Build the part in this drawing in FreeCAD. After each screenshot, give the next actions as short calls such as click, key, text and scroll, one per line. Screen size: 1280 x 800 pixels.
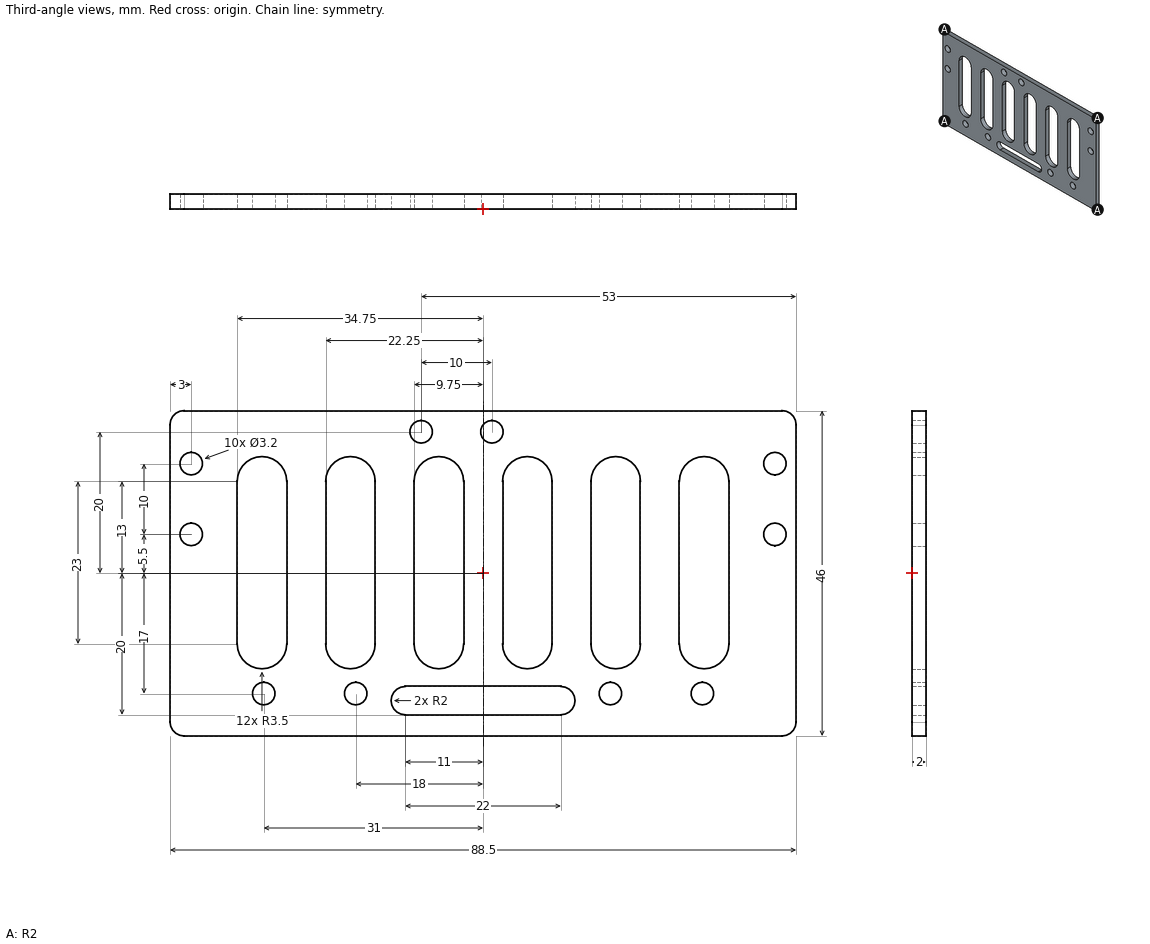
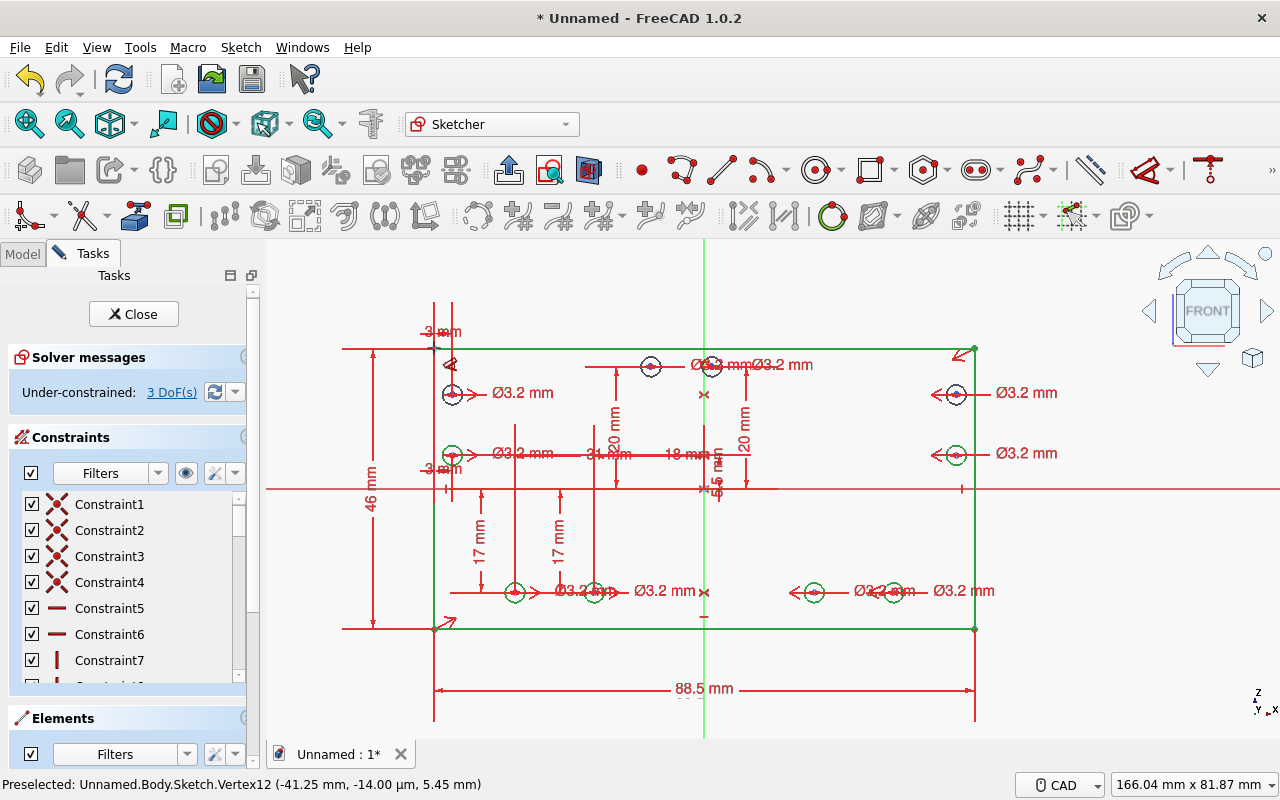
click(975, 349)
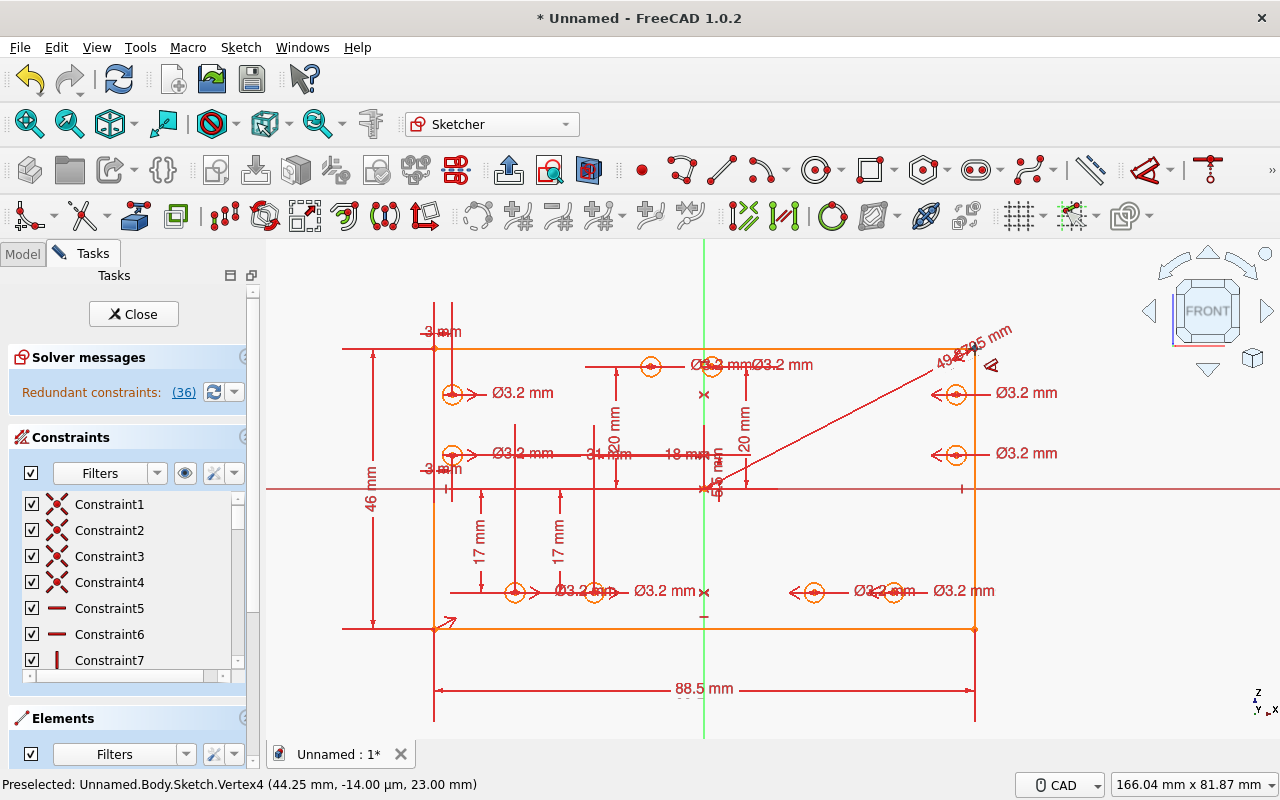
click(651, 367)
click(813, 315)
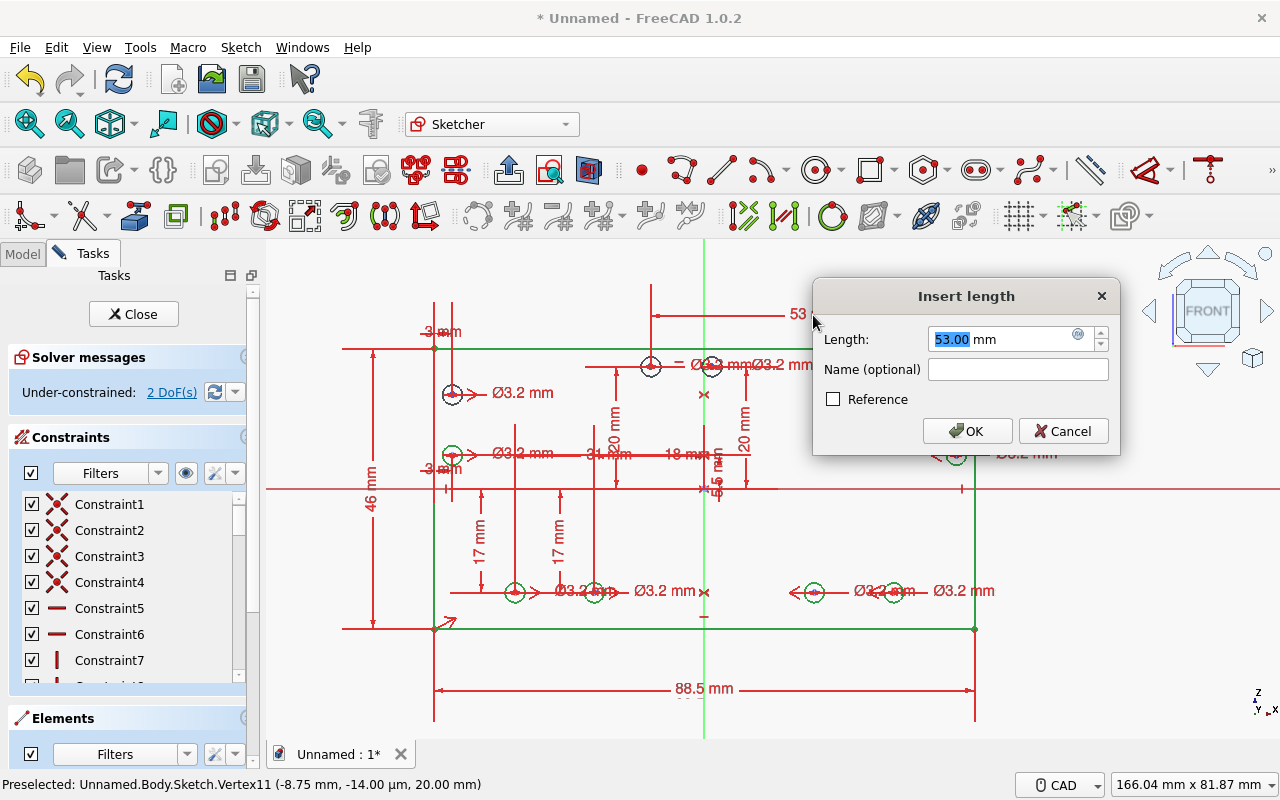
text(53)
key(Return)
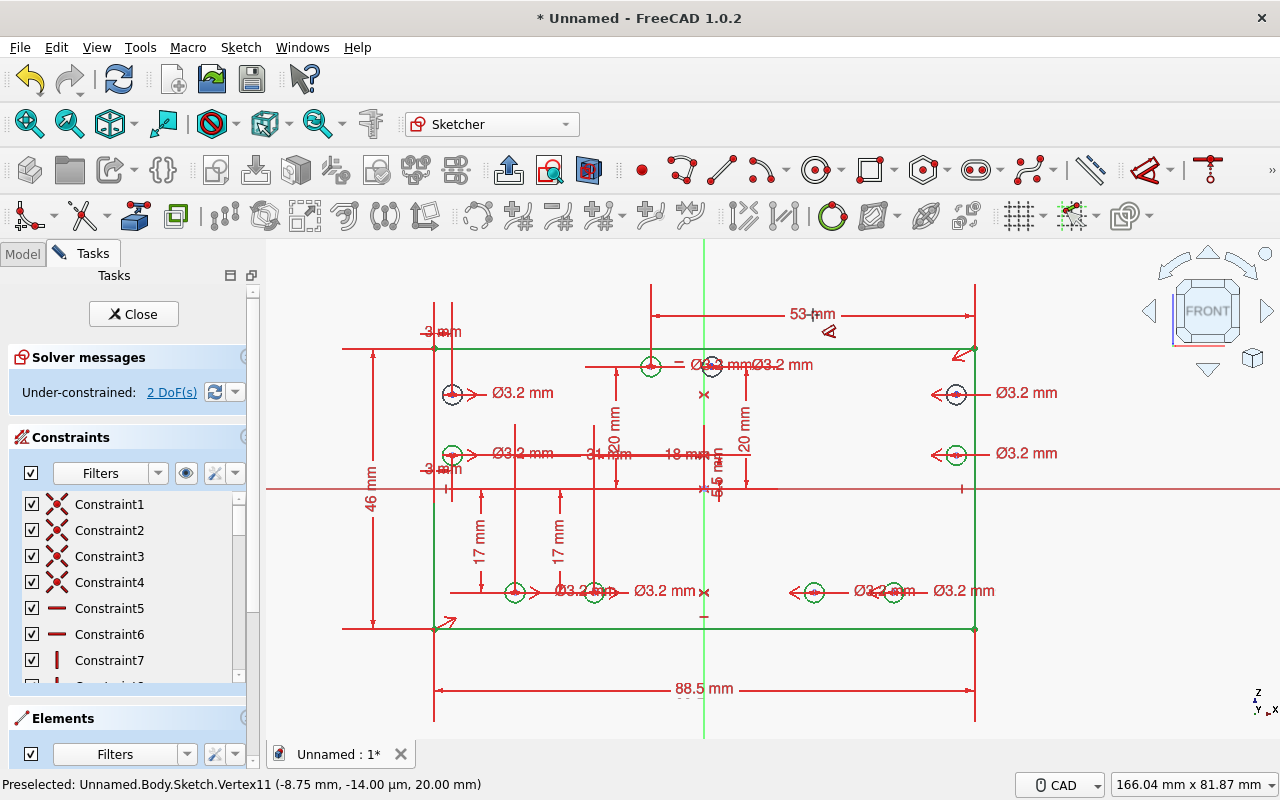
click(452, 395)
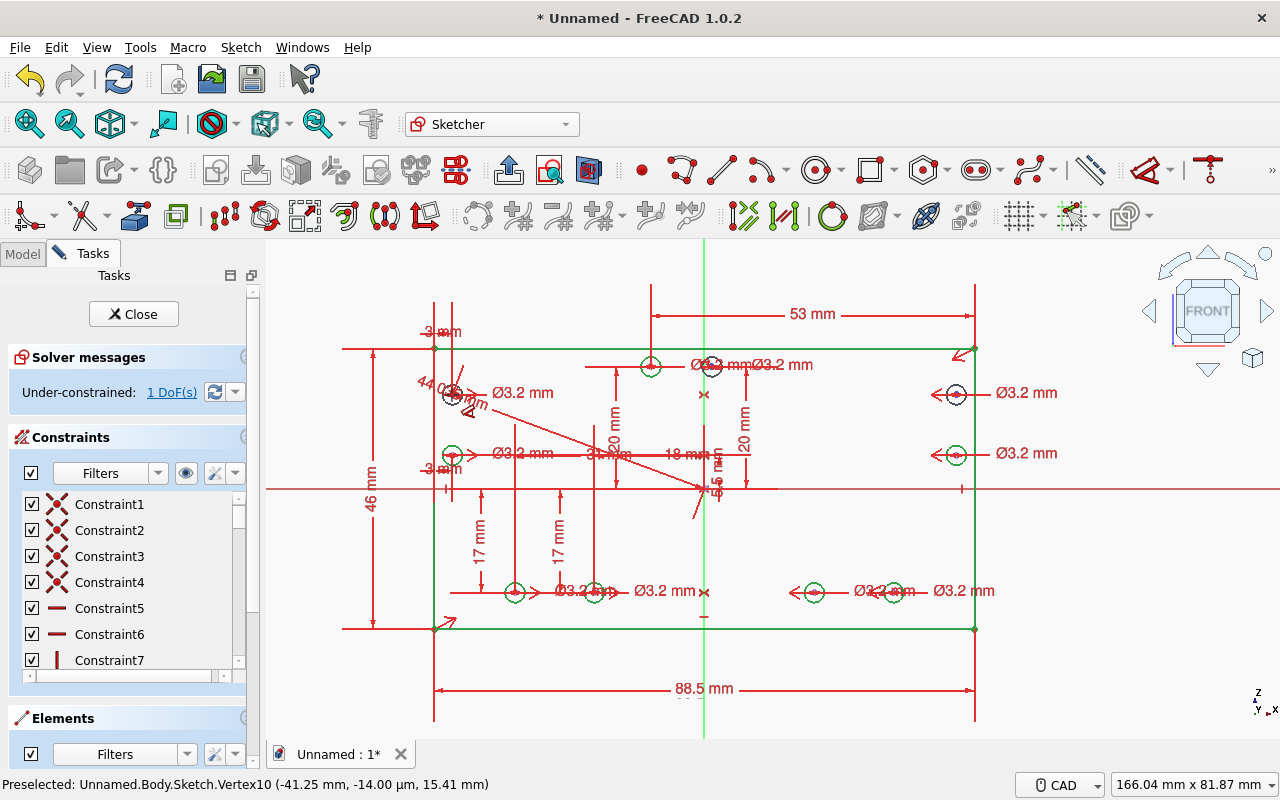
click(452, 455)
click(418, 425)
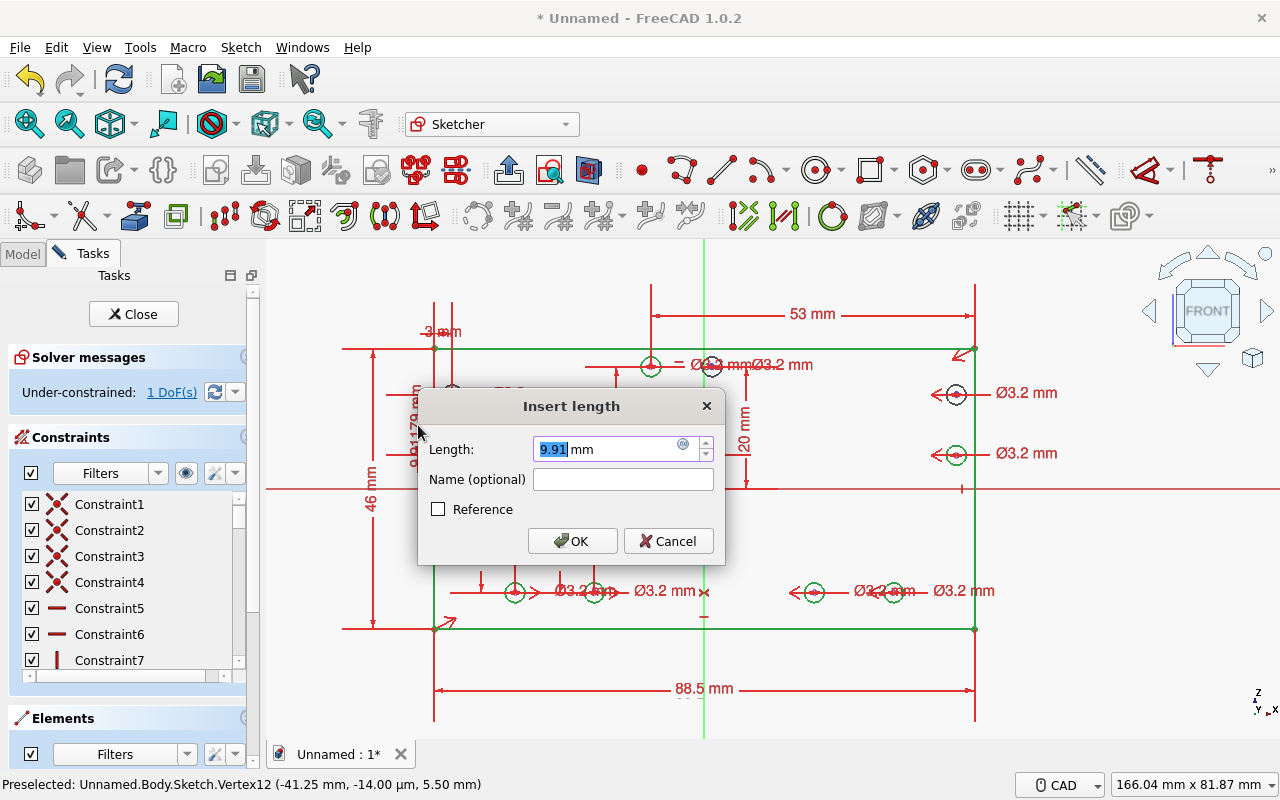
text(10)
key(Return)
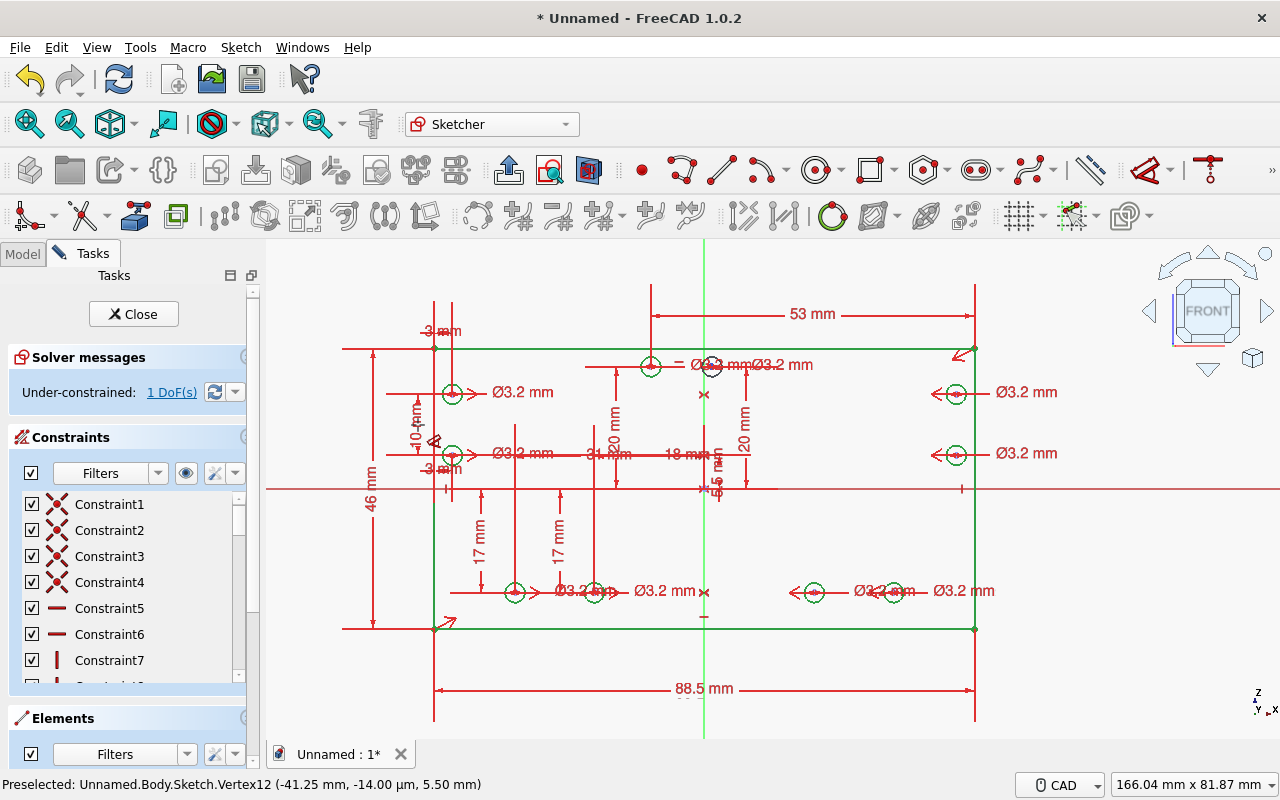
click(651, 367)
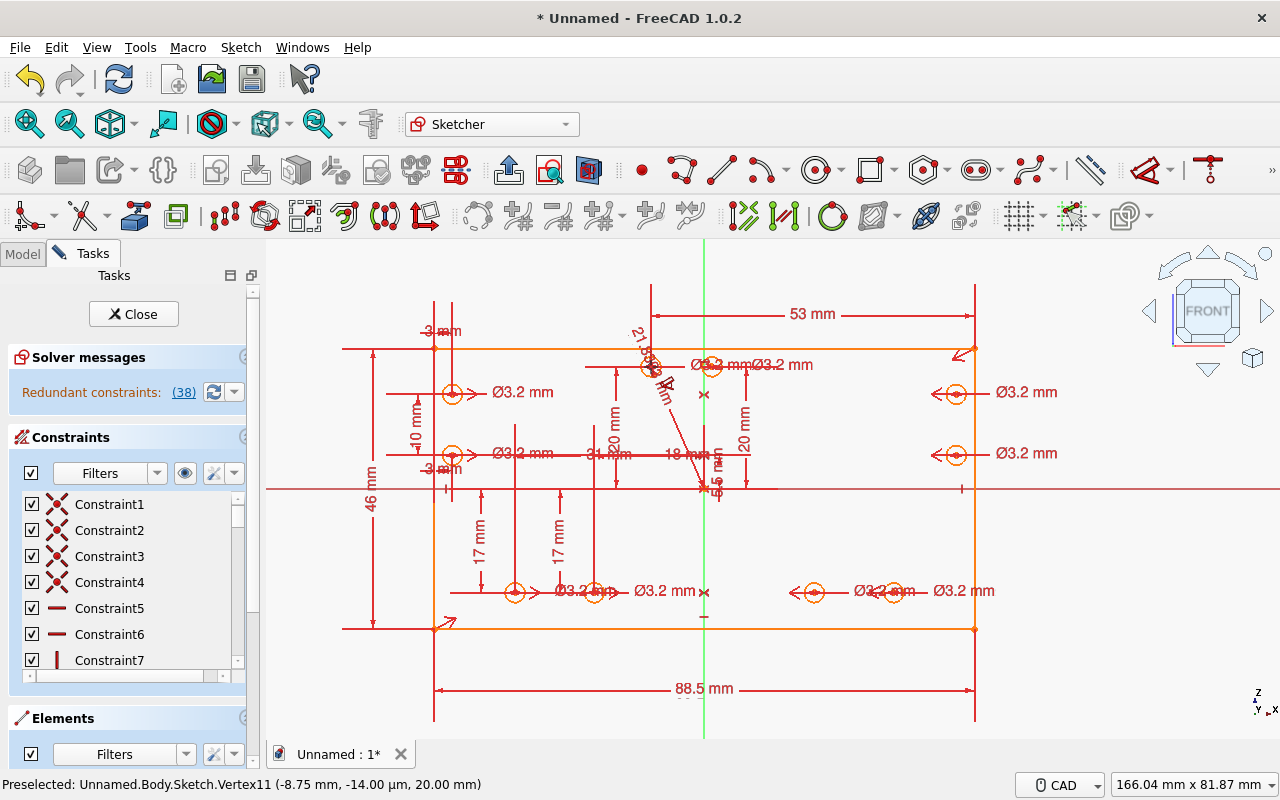
click(712, 367)
click(681, 333)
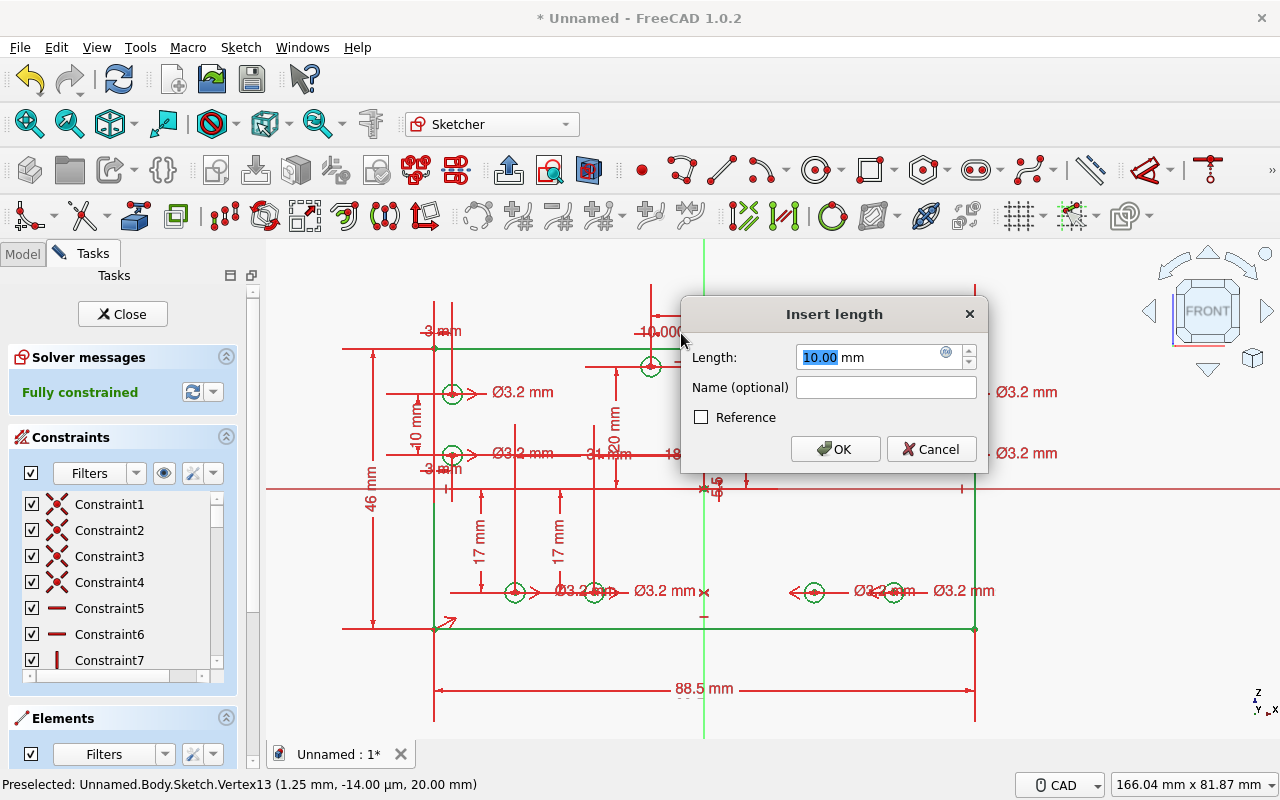
text(10)
key(Return)
key(Escape)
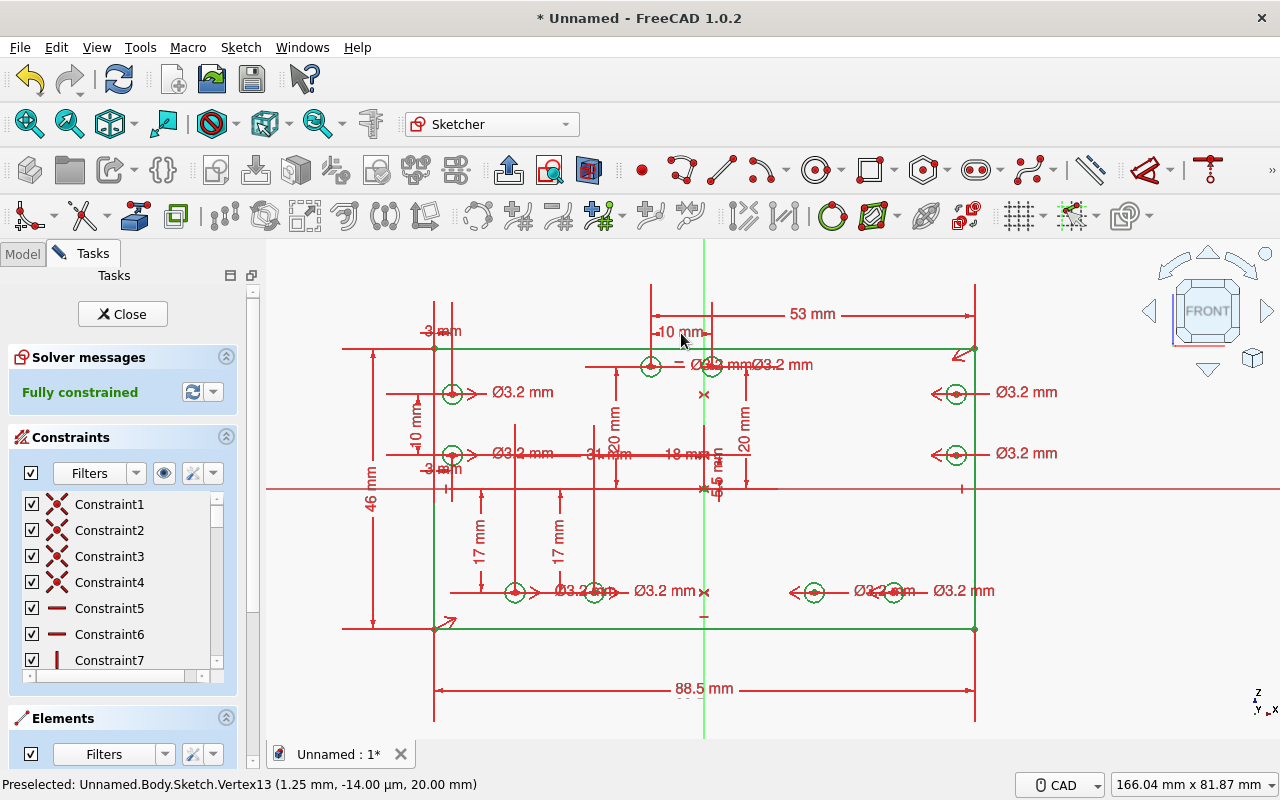
click(123, 314)